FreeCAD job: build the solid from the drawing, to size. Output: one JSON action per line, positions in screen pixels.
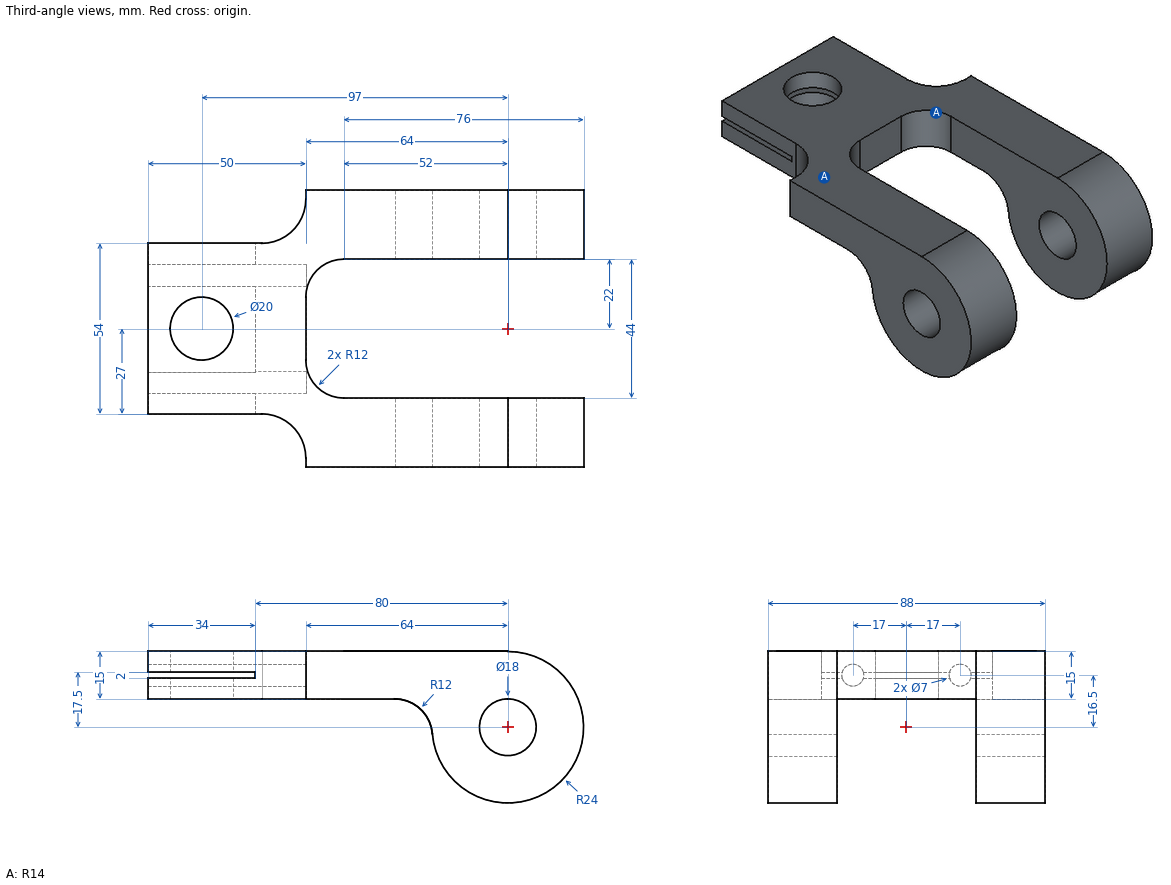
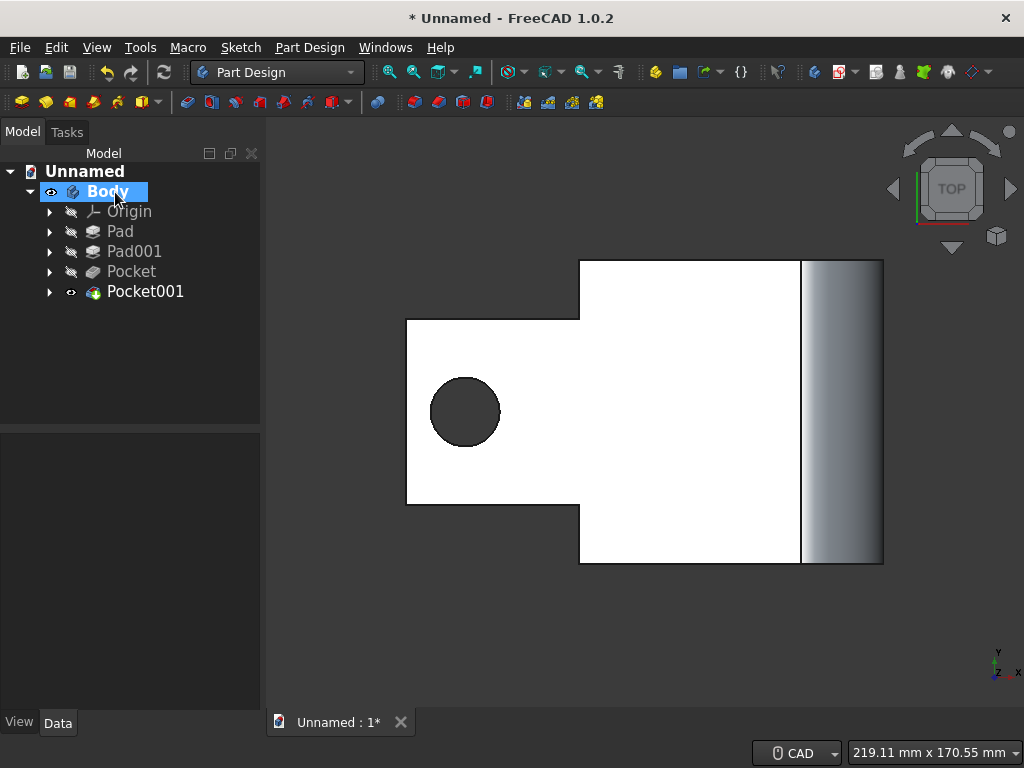
{"action": "key", "text": "0"}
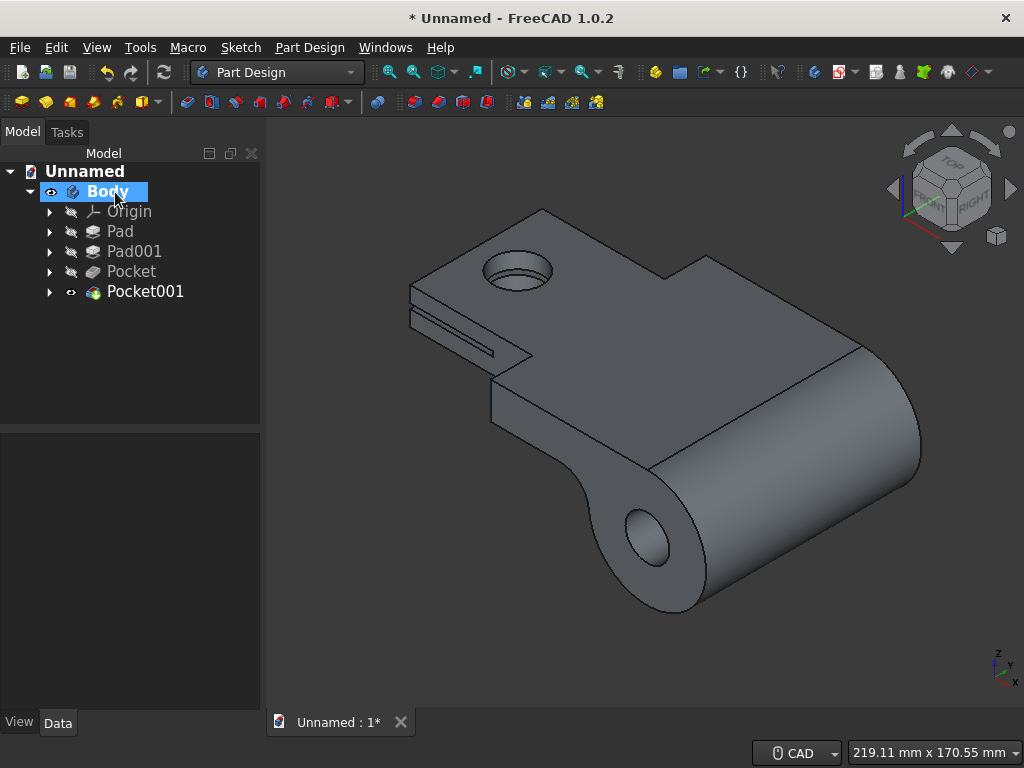
{"action": "key", "text": "1"}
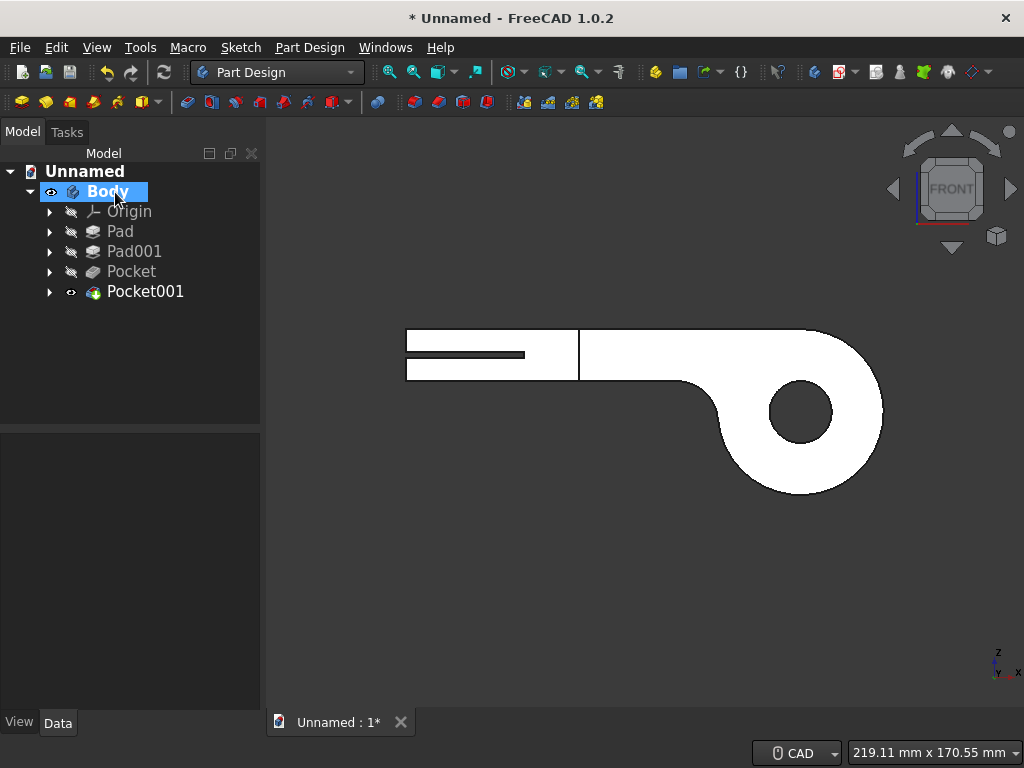
{"action": "key", "text": "3"}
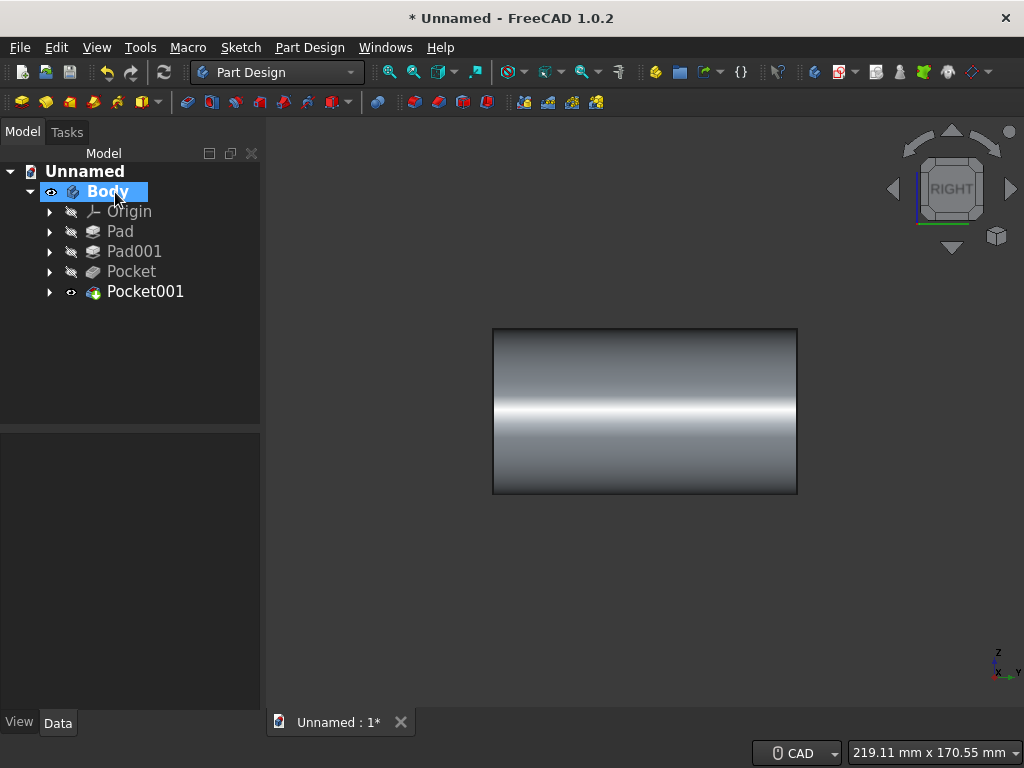
{"action": "left_click", "coordinate": [390, 72]}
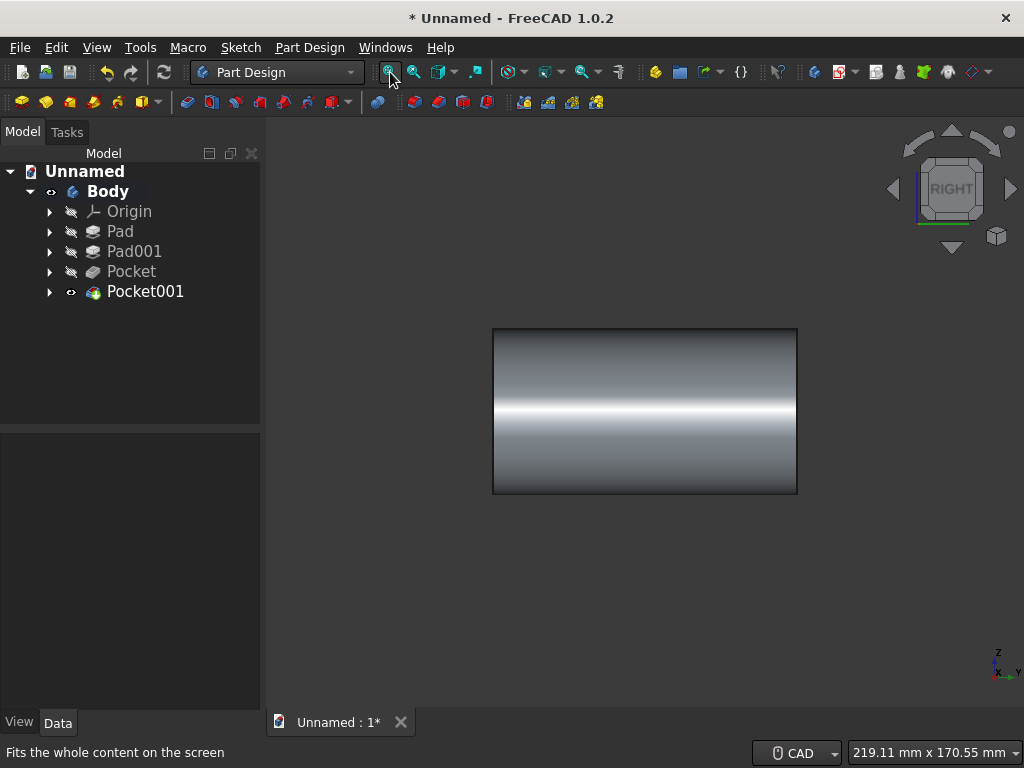
{"action": "key", "text": "5"}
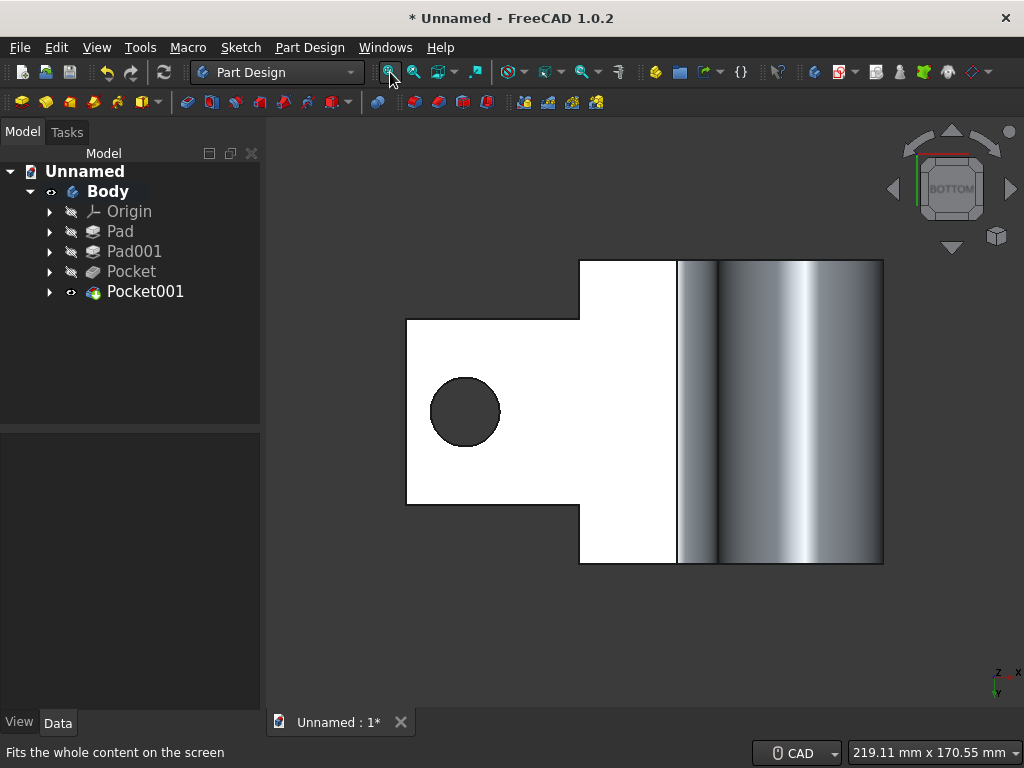
{"action": "key", "text": "4"}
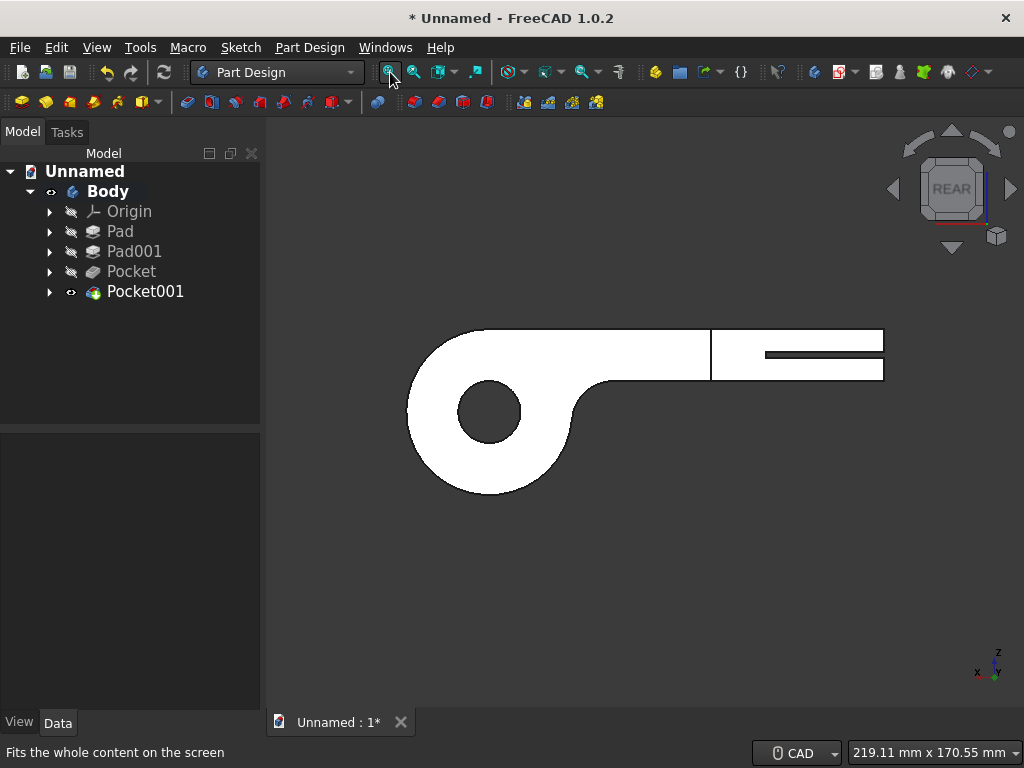
{"action": "key", "text": "6"}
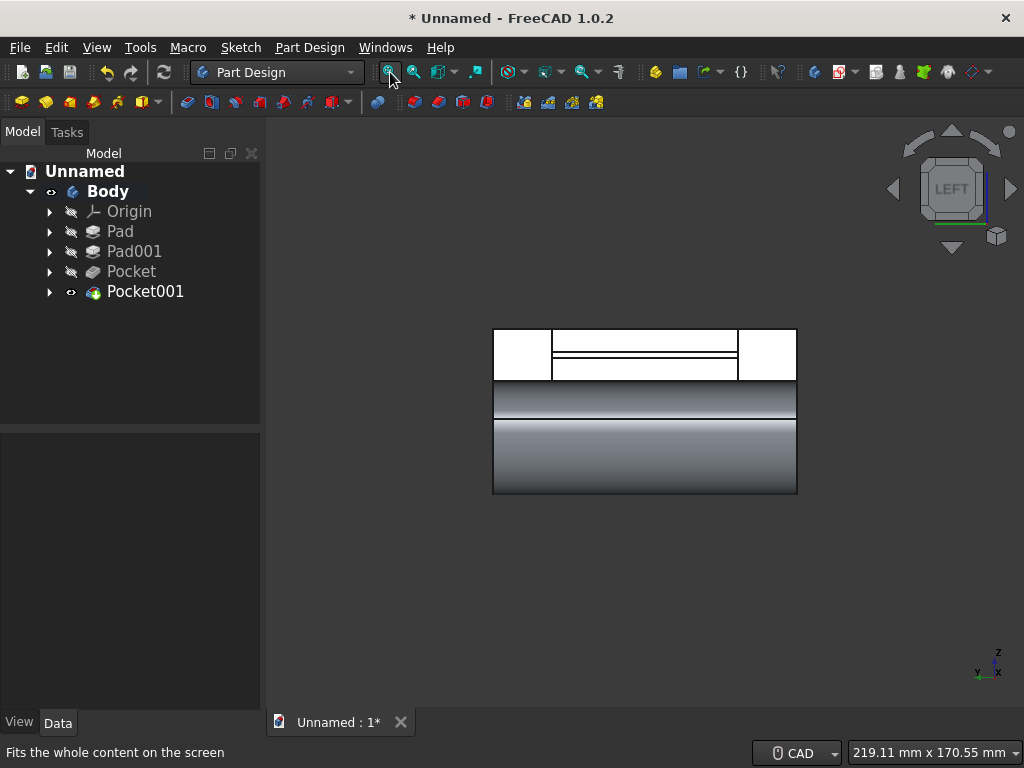
{"action": "left_click", "coordinate": [390, 72]}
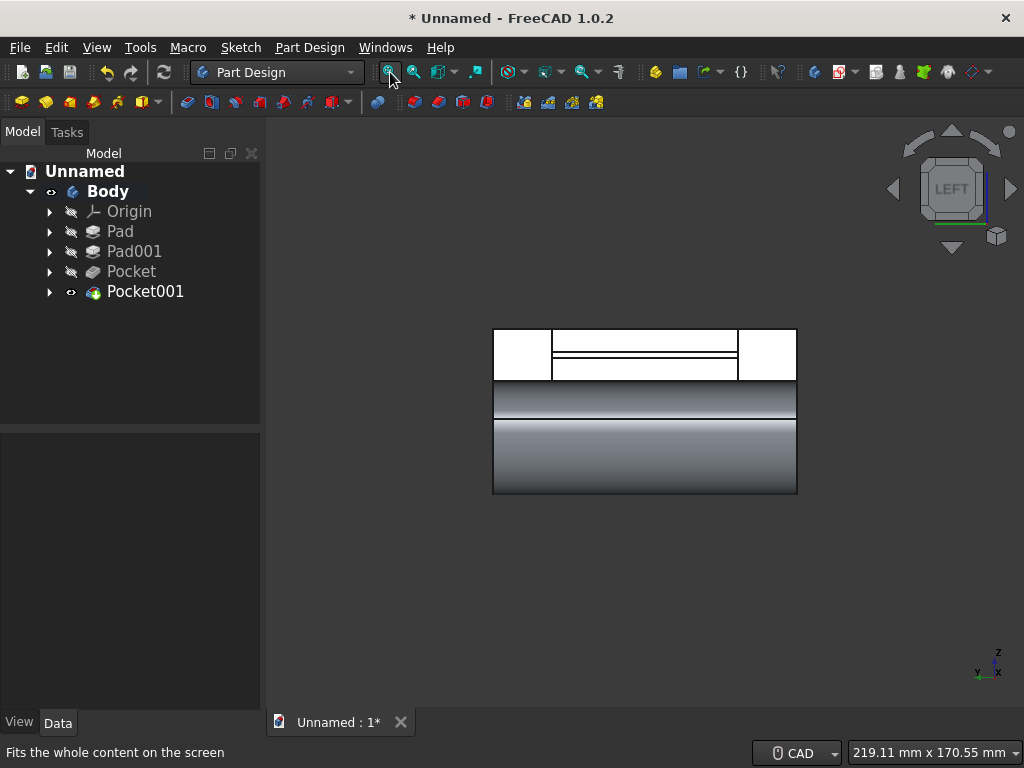
{"action": "key", "text": "v 3"}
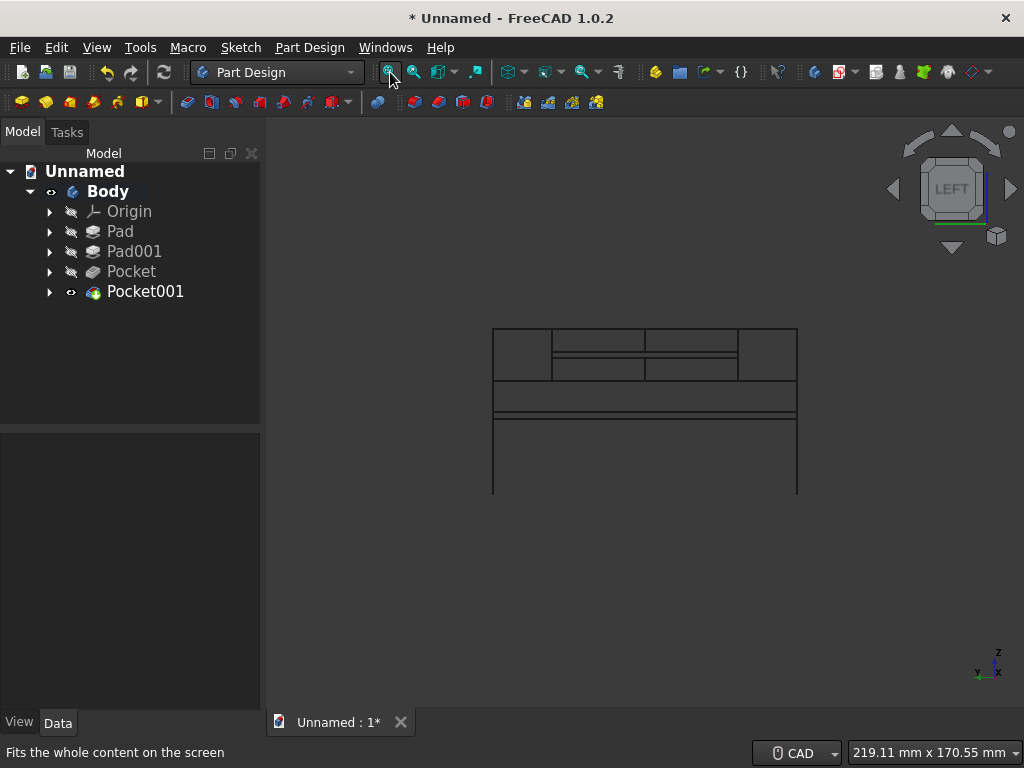
{"action": "key", "text": "0"}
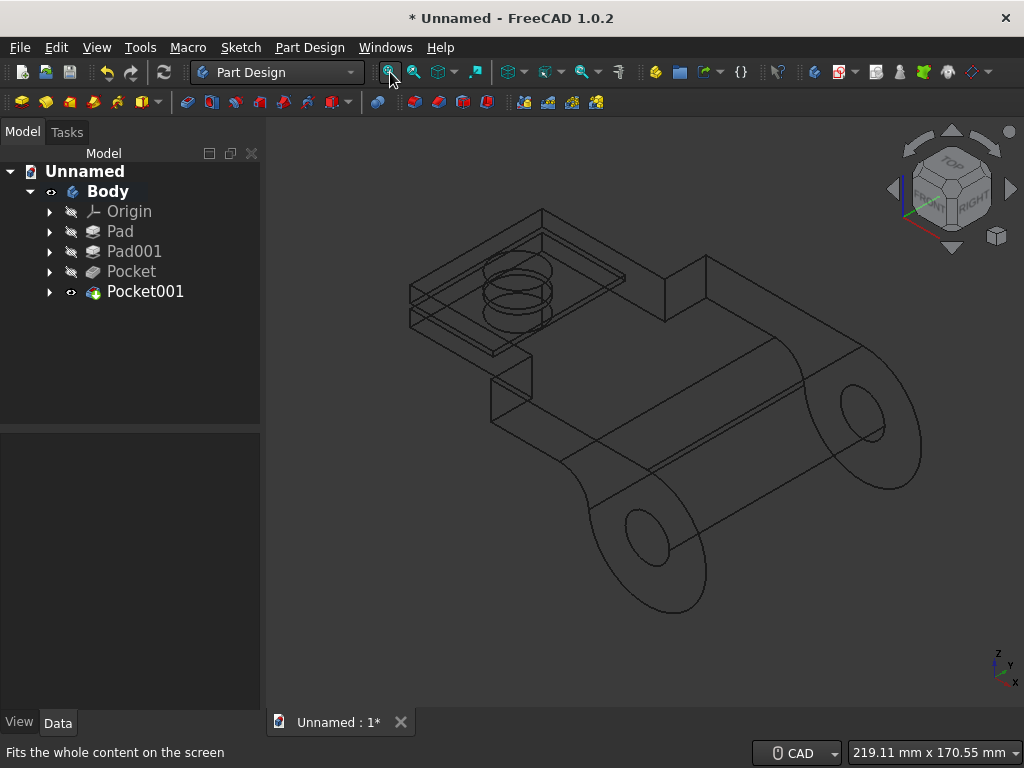
{"action": "left_click", "coordinate": [532, 376]}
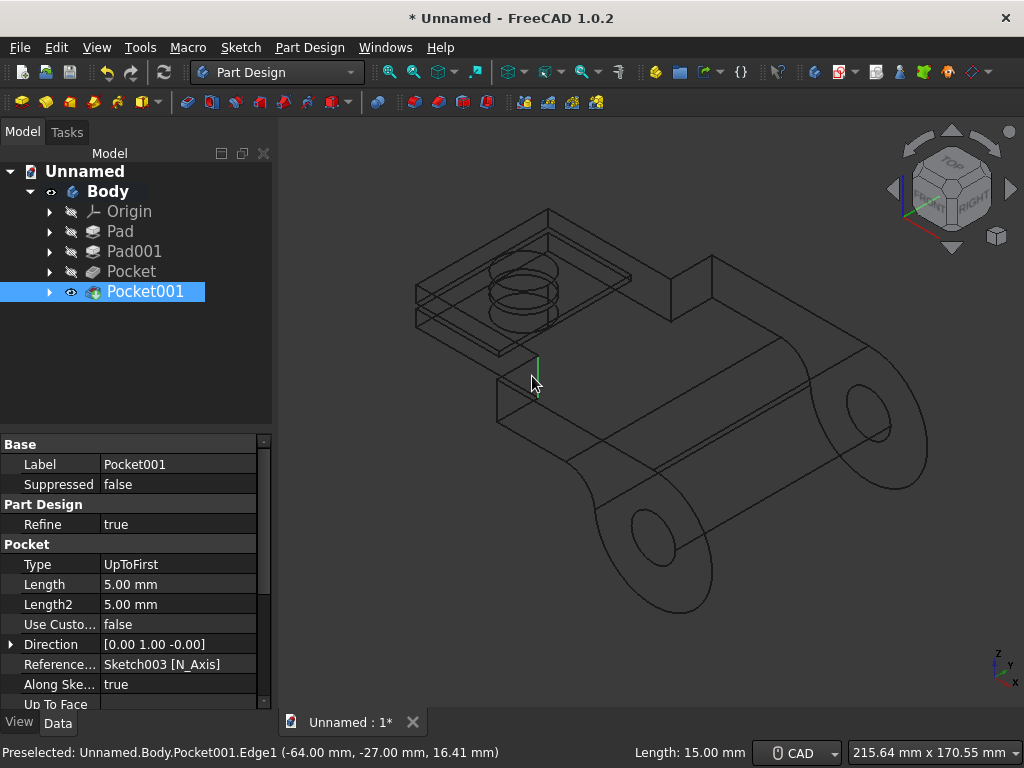
{"action": "left_click", "coordinate": [671, 299], "text": "ctrl"}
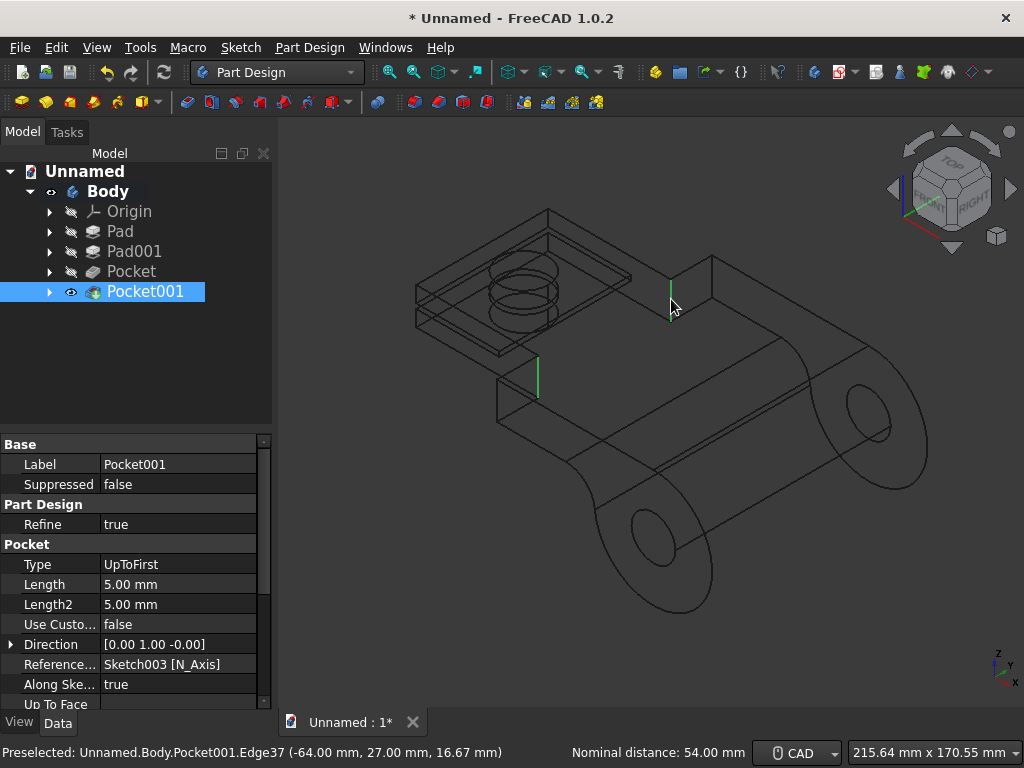
{"action": "key", "text": "v 1"}